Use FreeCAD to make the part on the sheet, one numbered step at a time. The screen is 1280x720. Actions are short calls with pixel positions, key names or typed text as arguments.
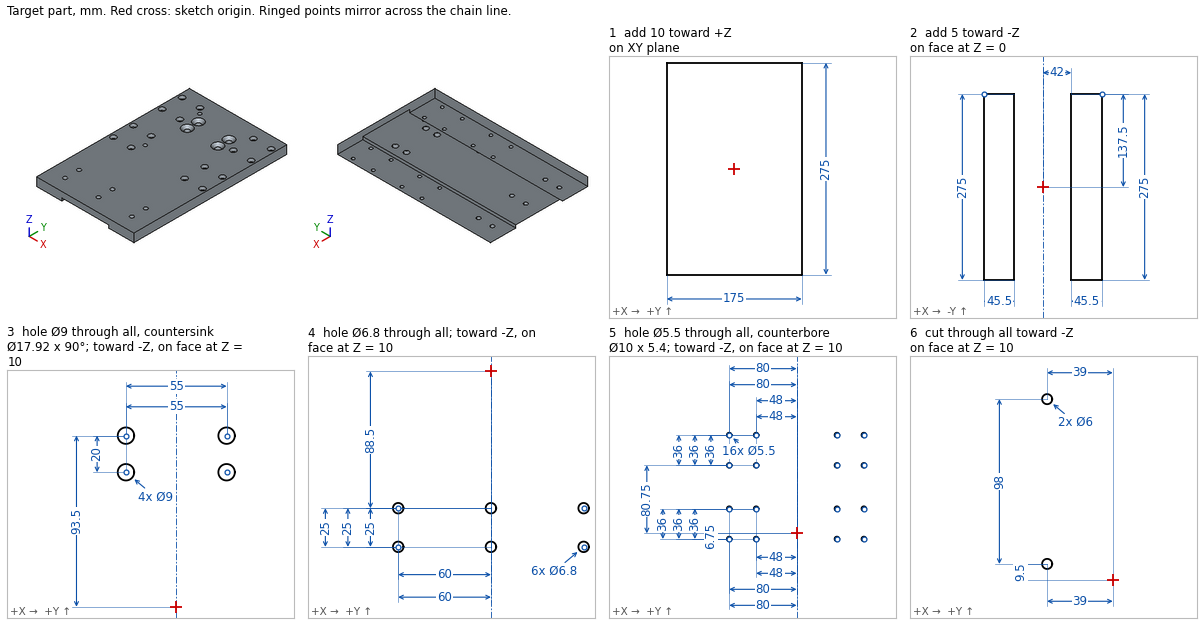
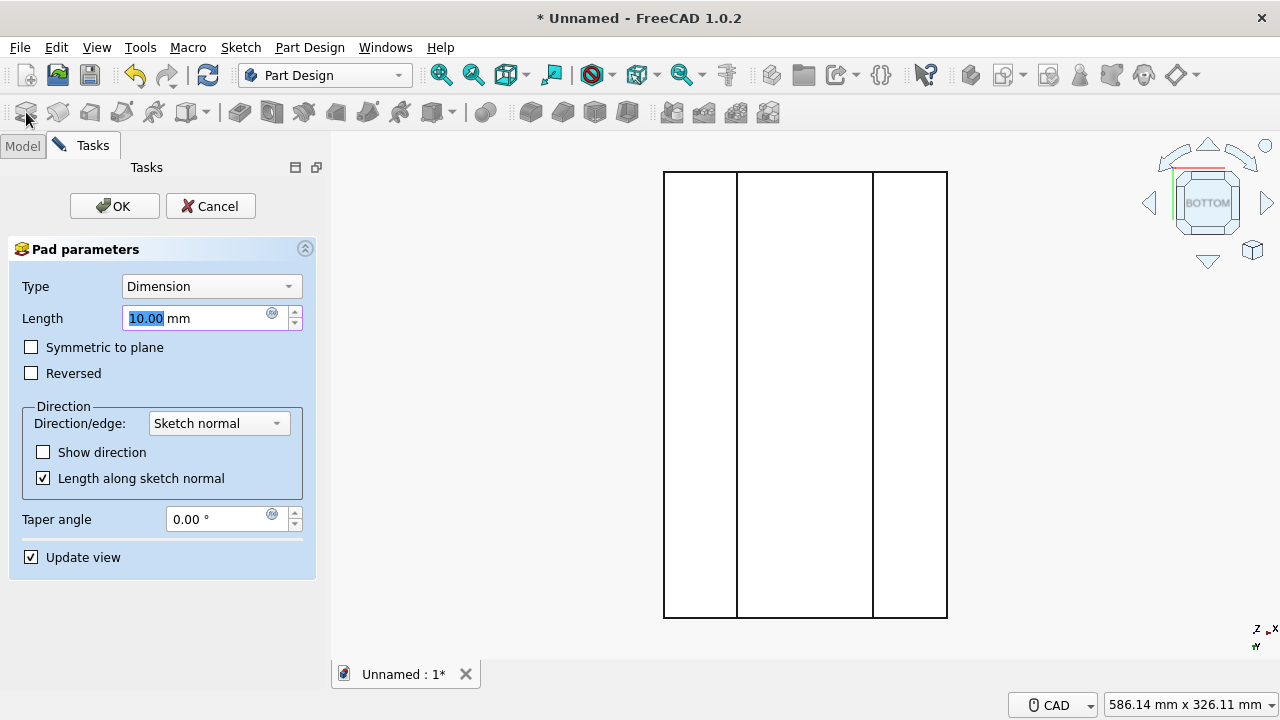
text(5)
key(Tab)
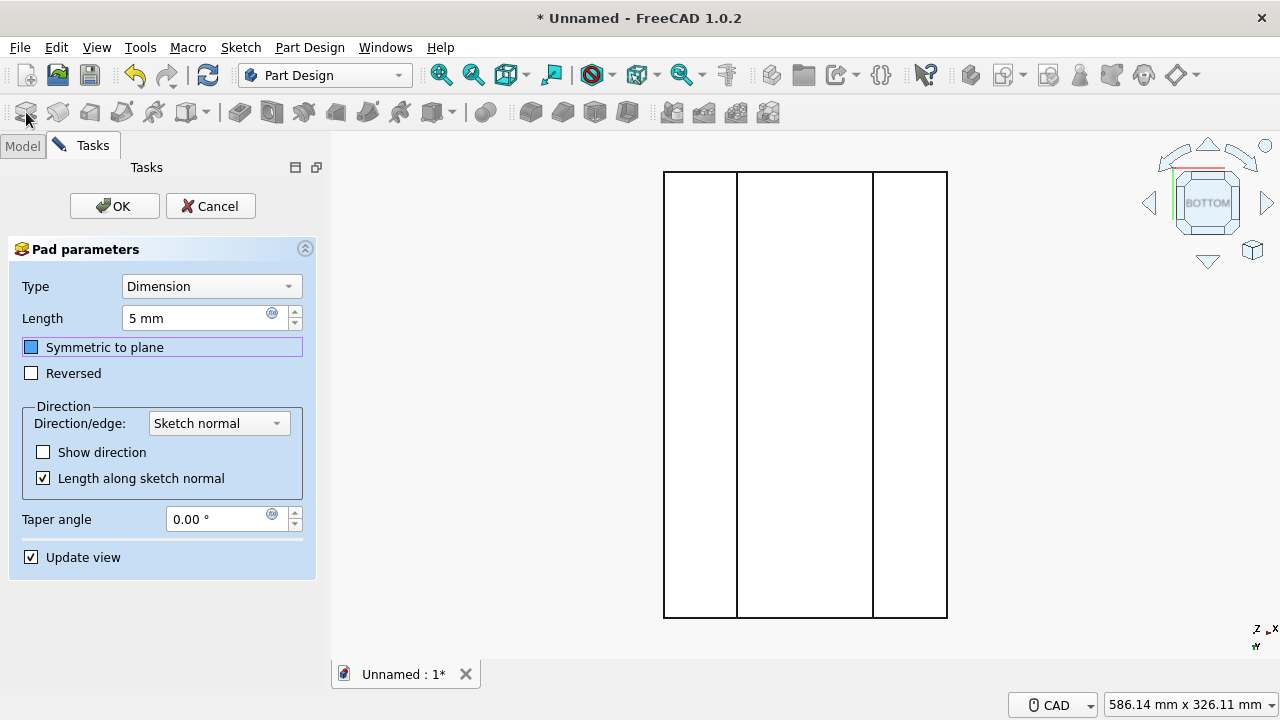
click(115, 206)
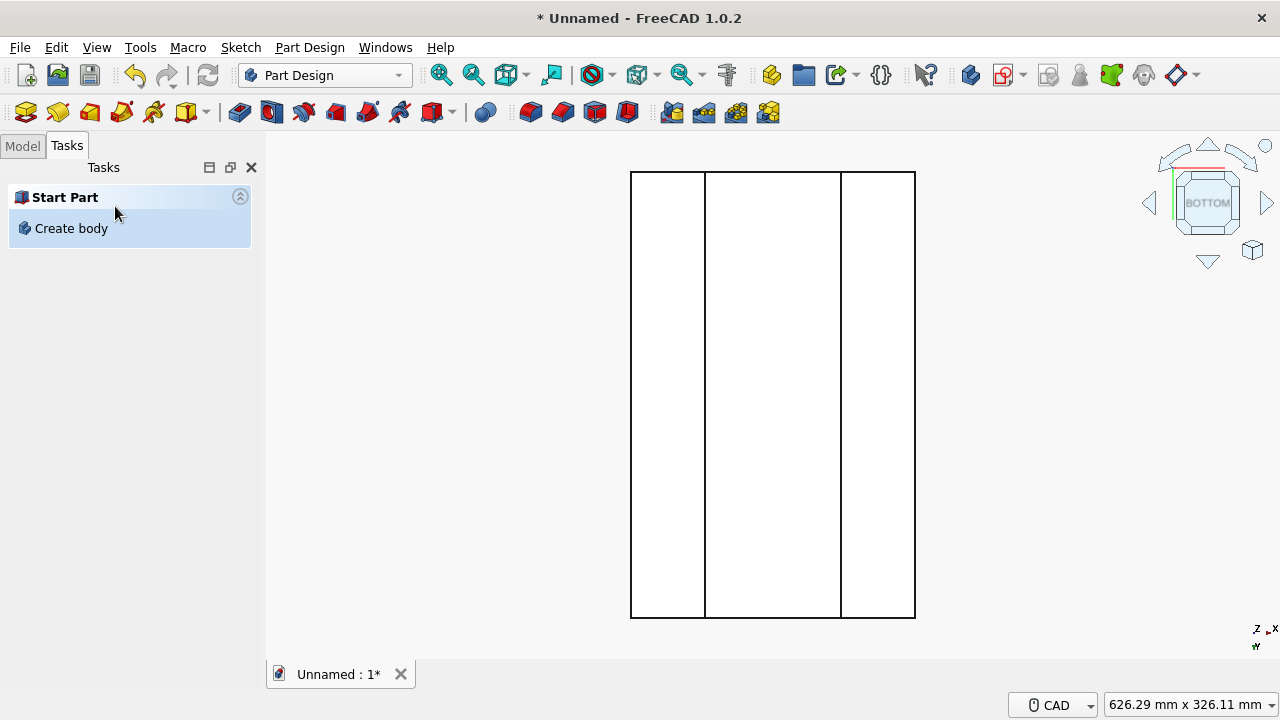
key(0)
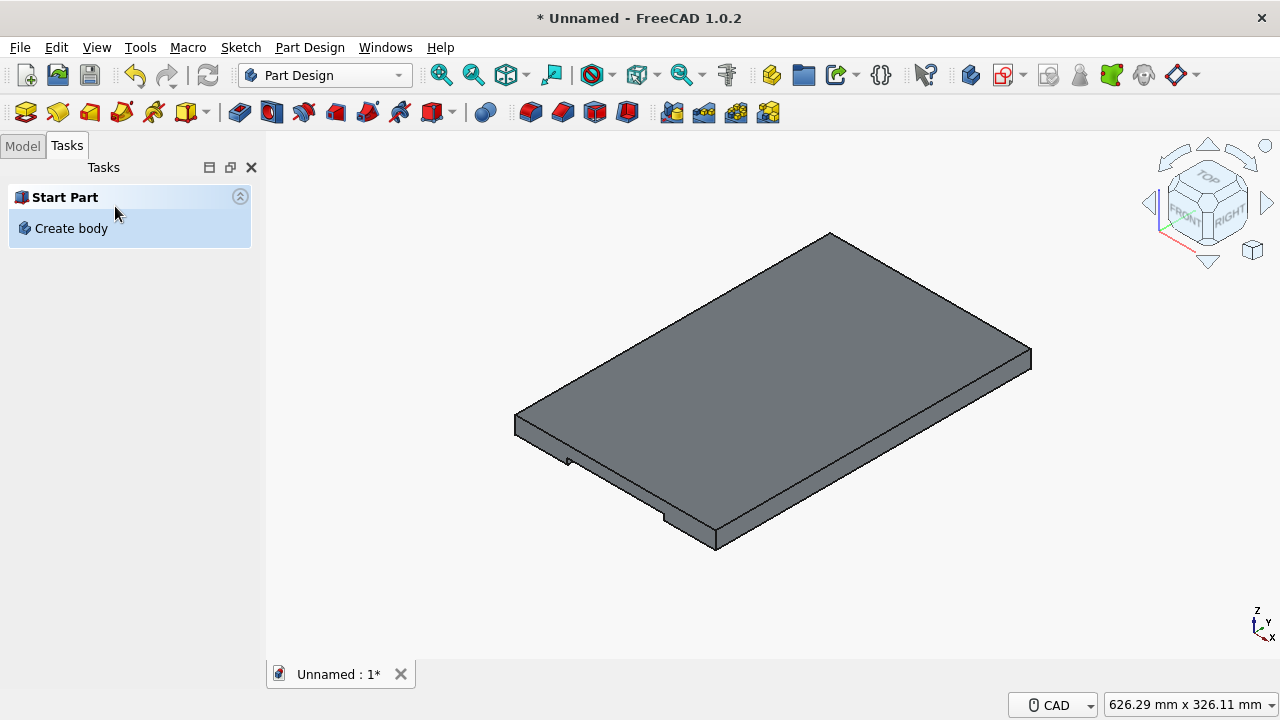
click(818, 355)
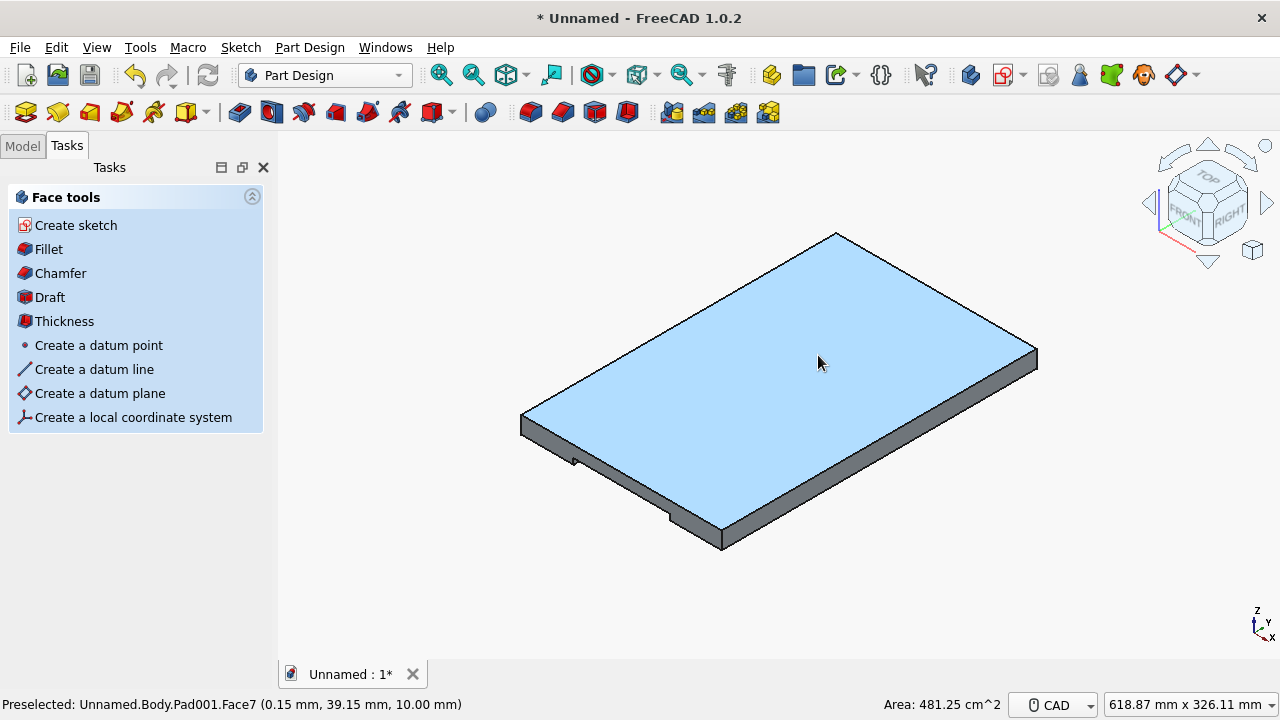
click(1004, 76)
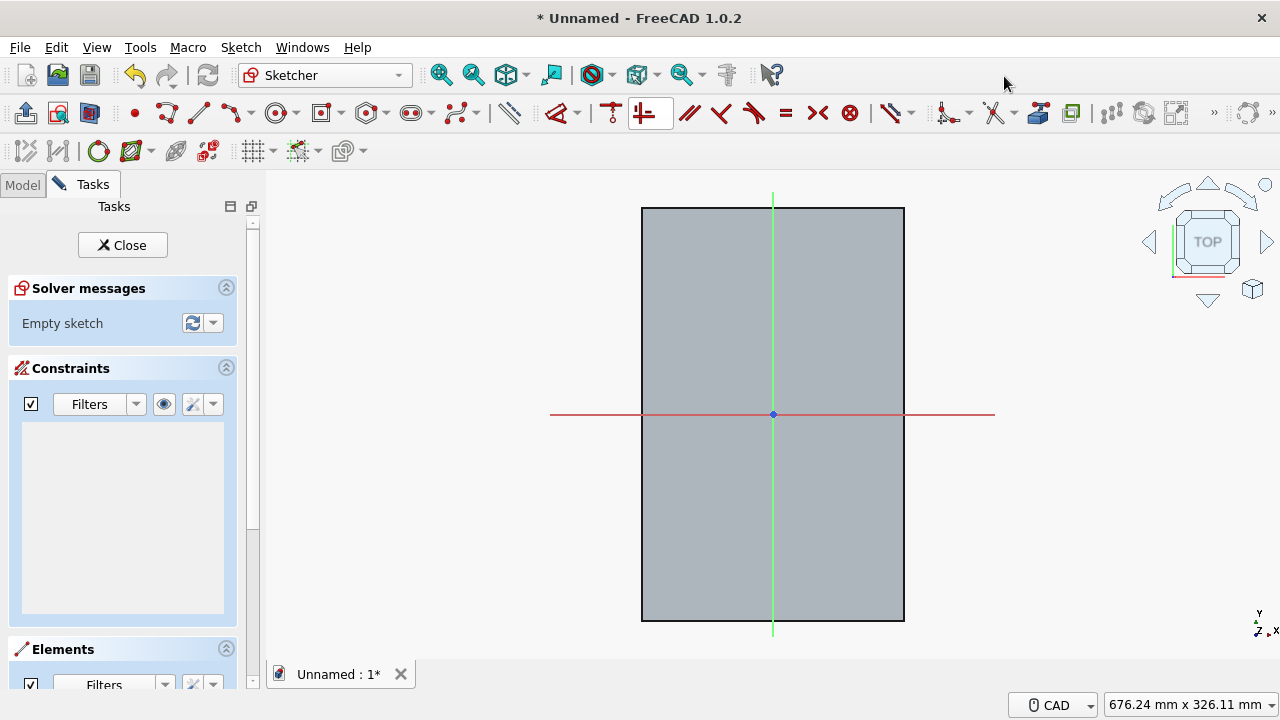
scroll(829, 281, up, 4)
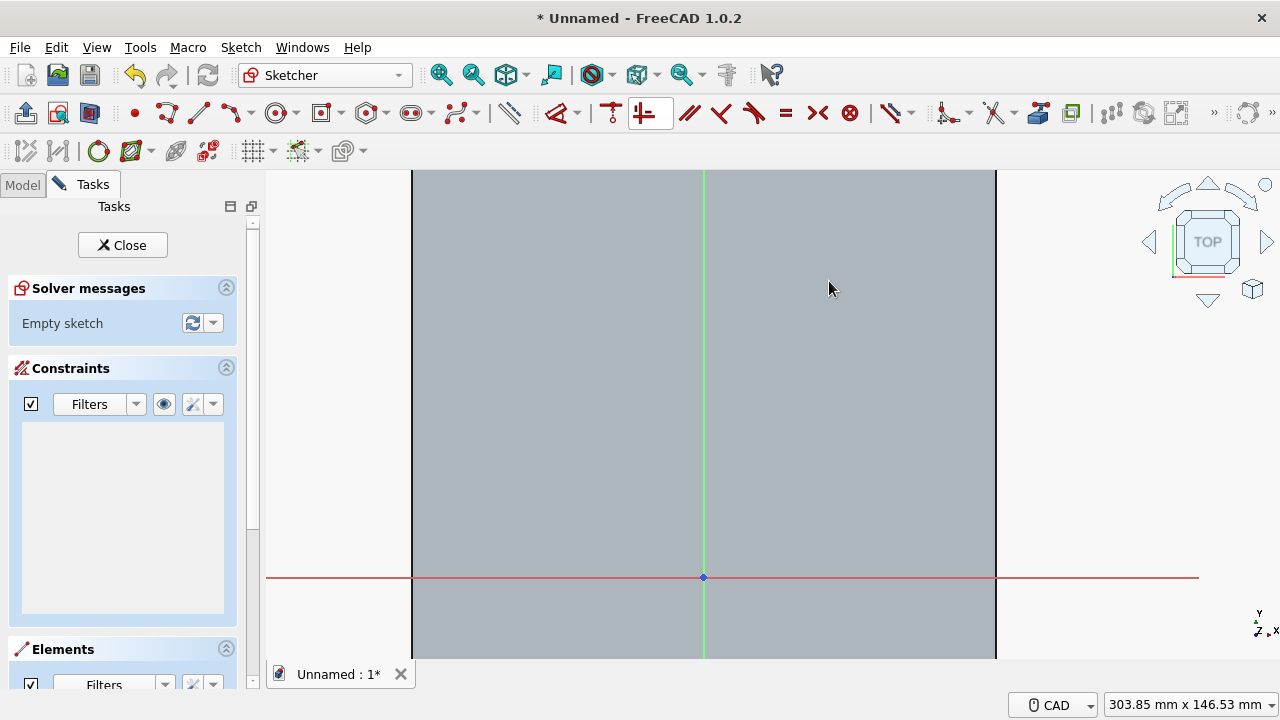
key(g)
key(c)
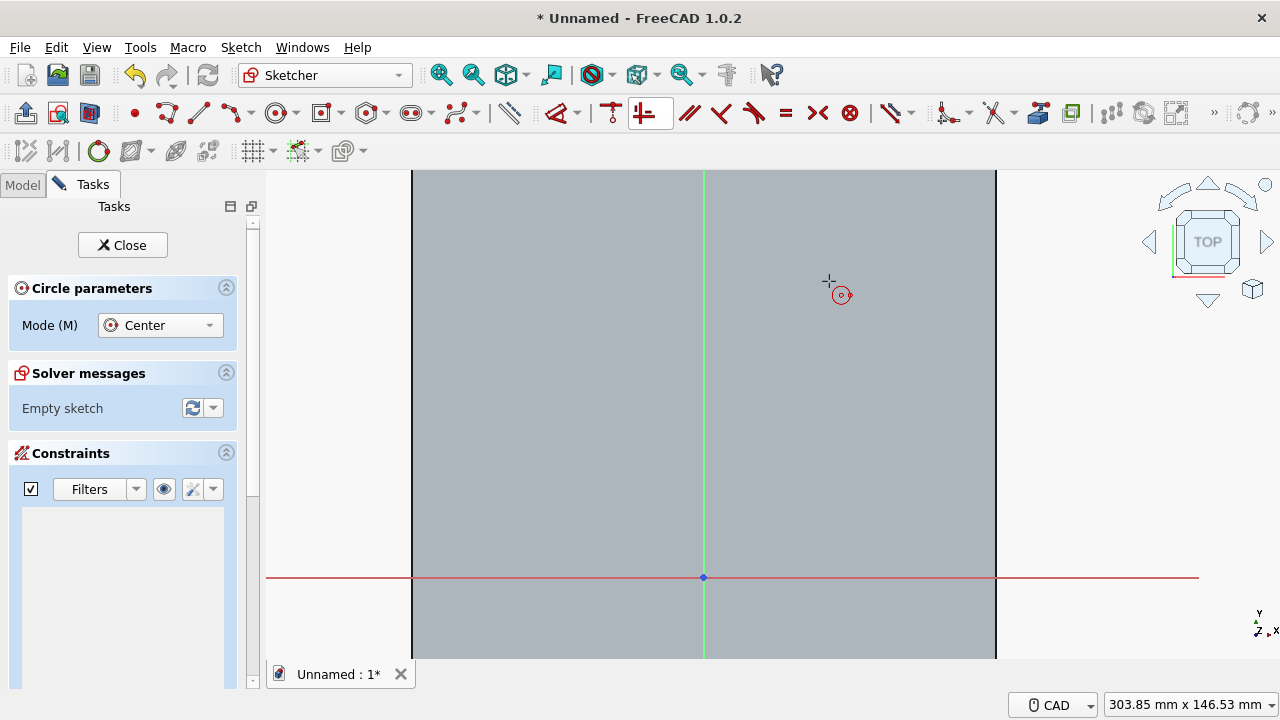
scroll(612, 266, up, 3)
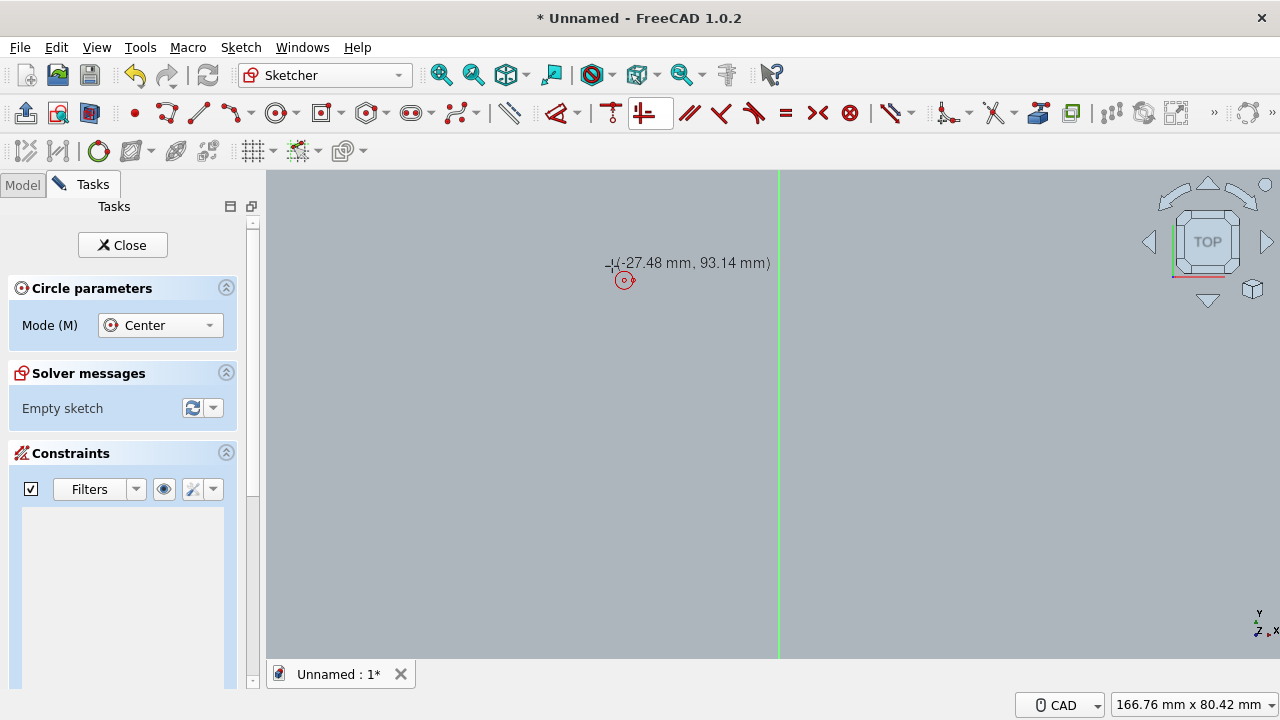
click(612, 265)
move(631, 246)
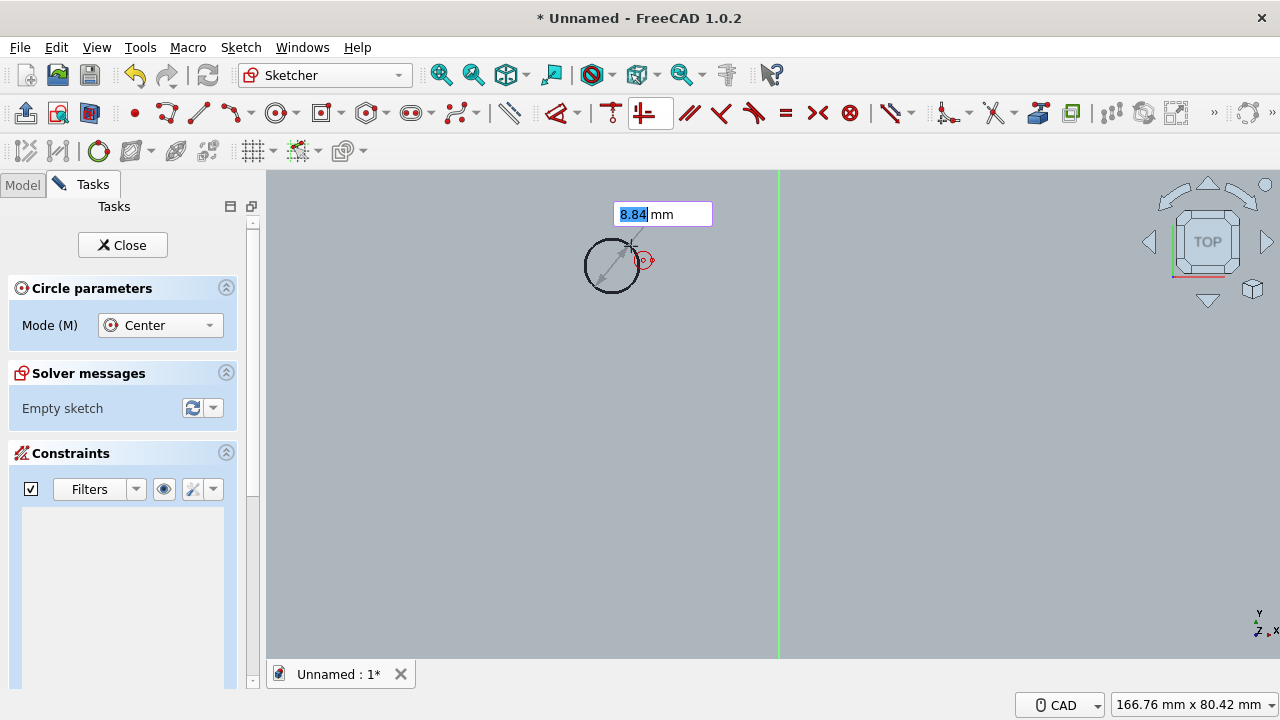
text(9)
key(Return)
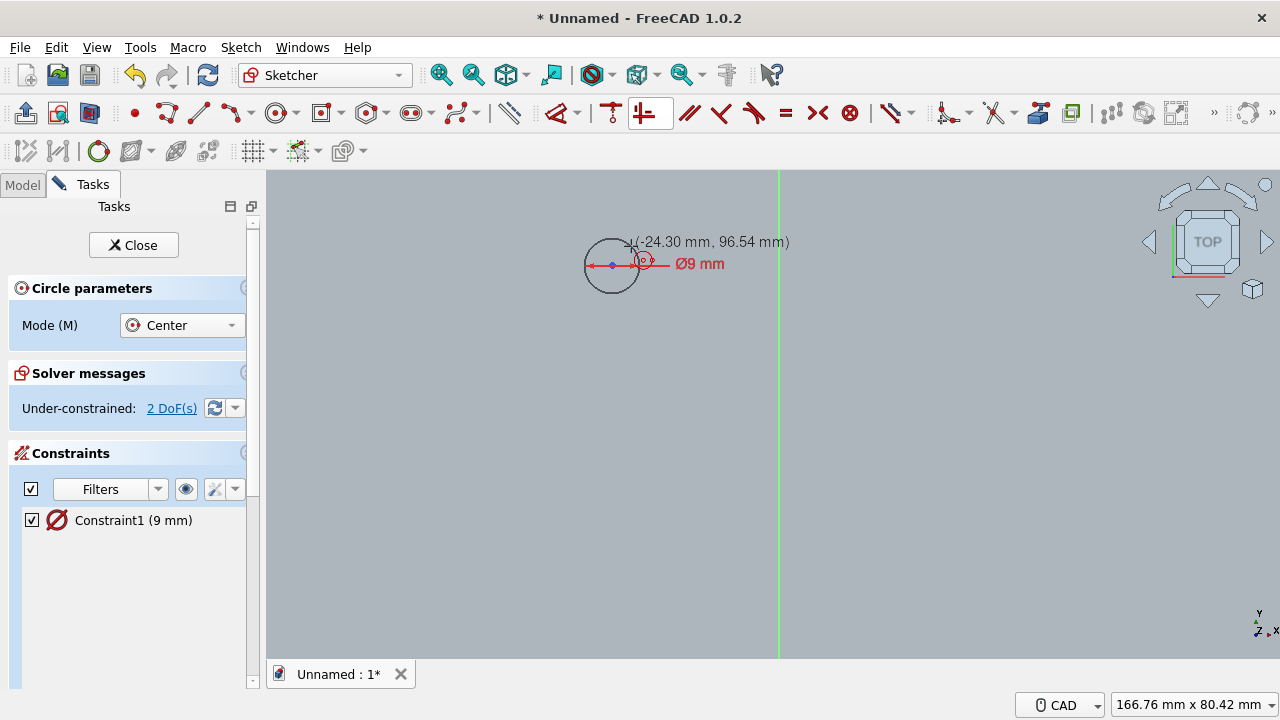
click(612, 387)
move(631, 368)